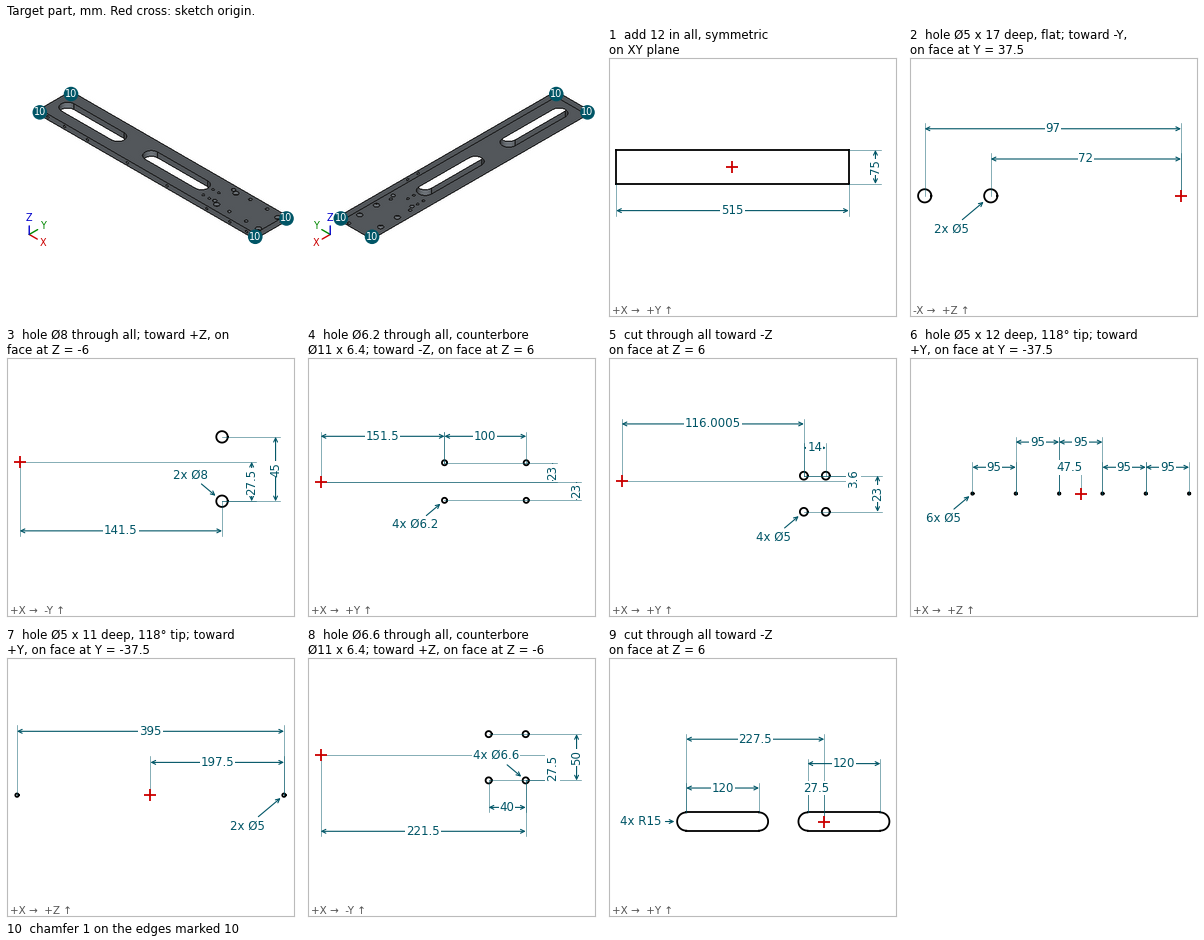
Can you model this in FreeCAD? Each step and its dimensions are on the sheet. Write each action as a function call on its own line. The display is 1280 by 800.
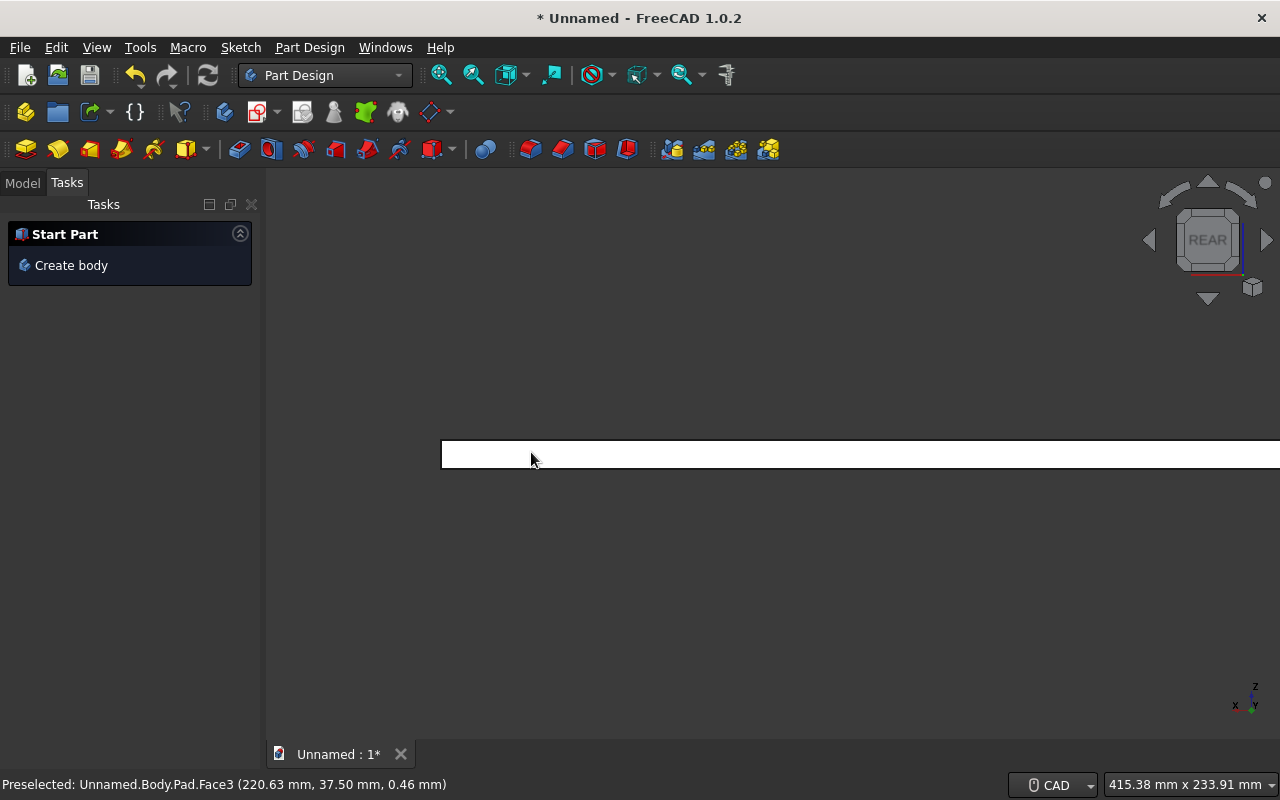
click(530, 454)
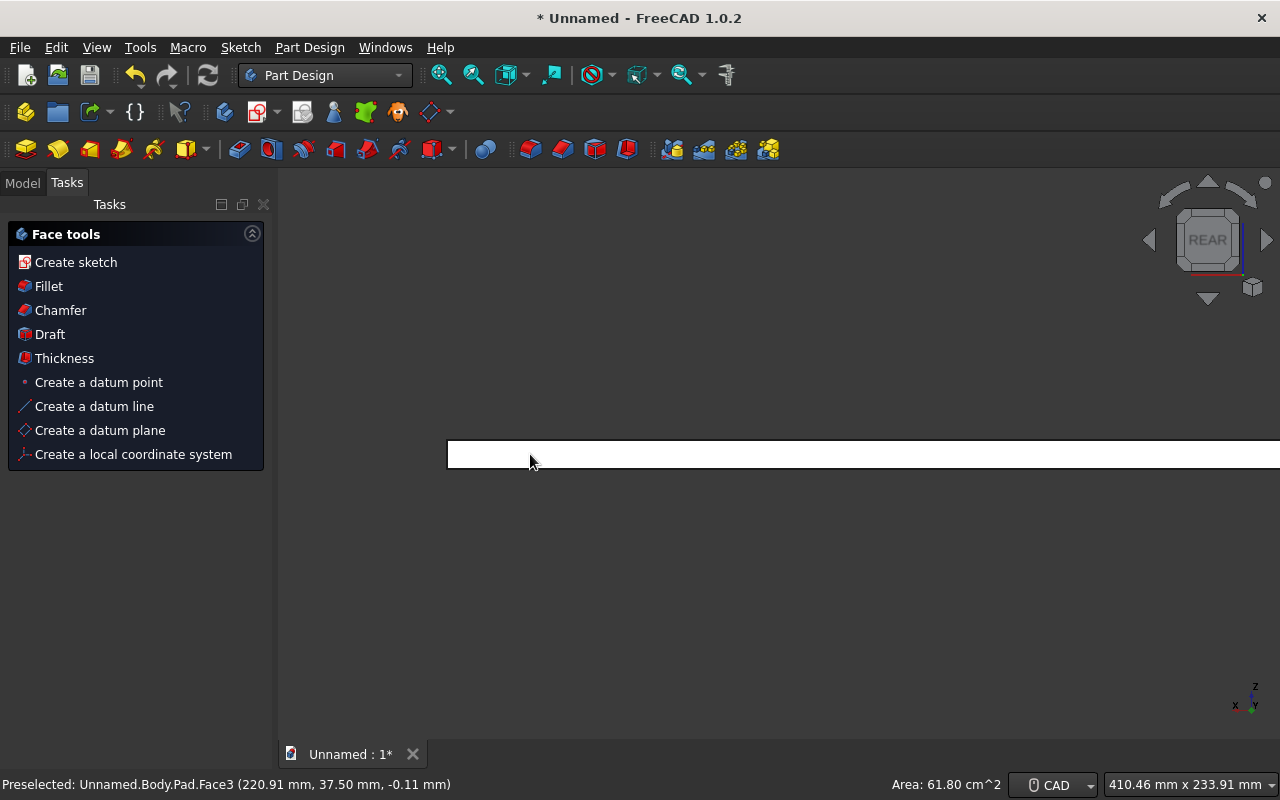
click(258, 112)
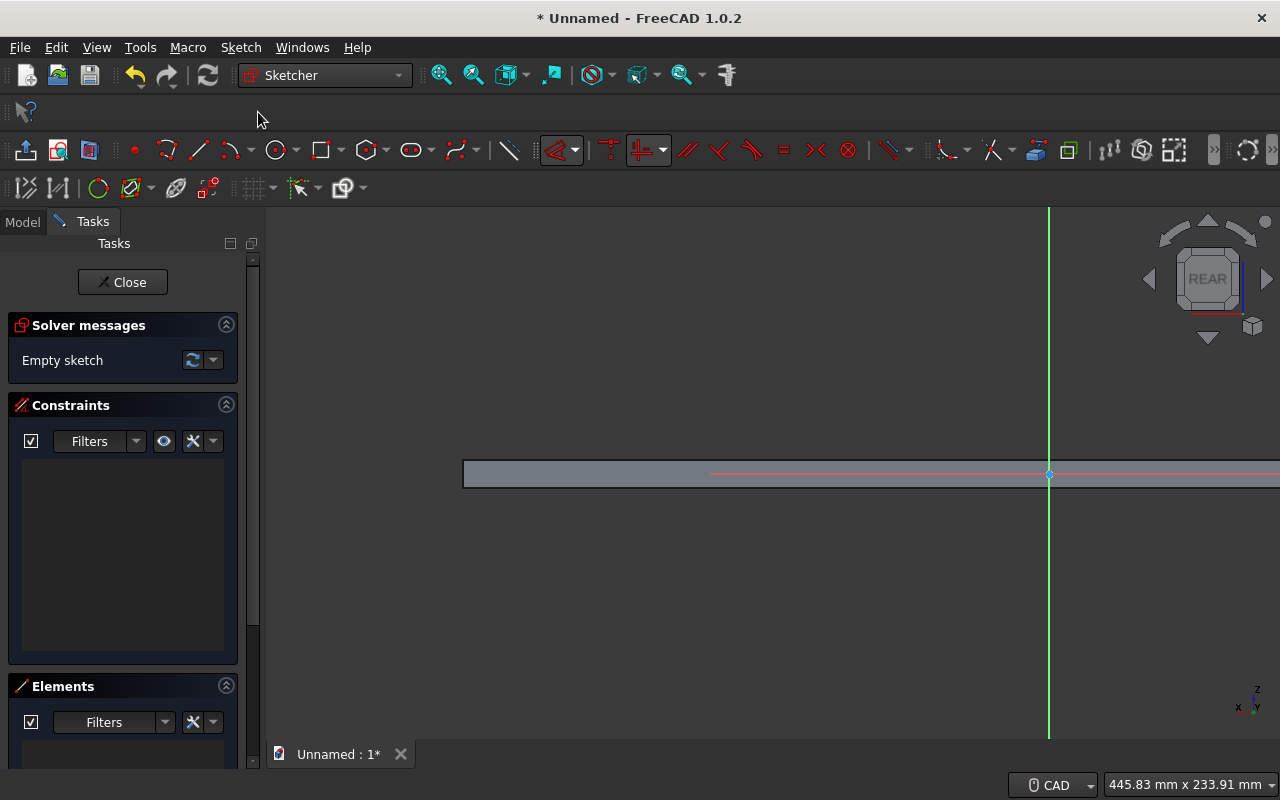
scroll(876, 474, up, 11)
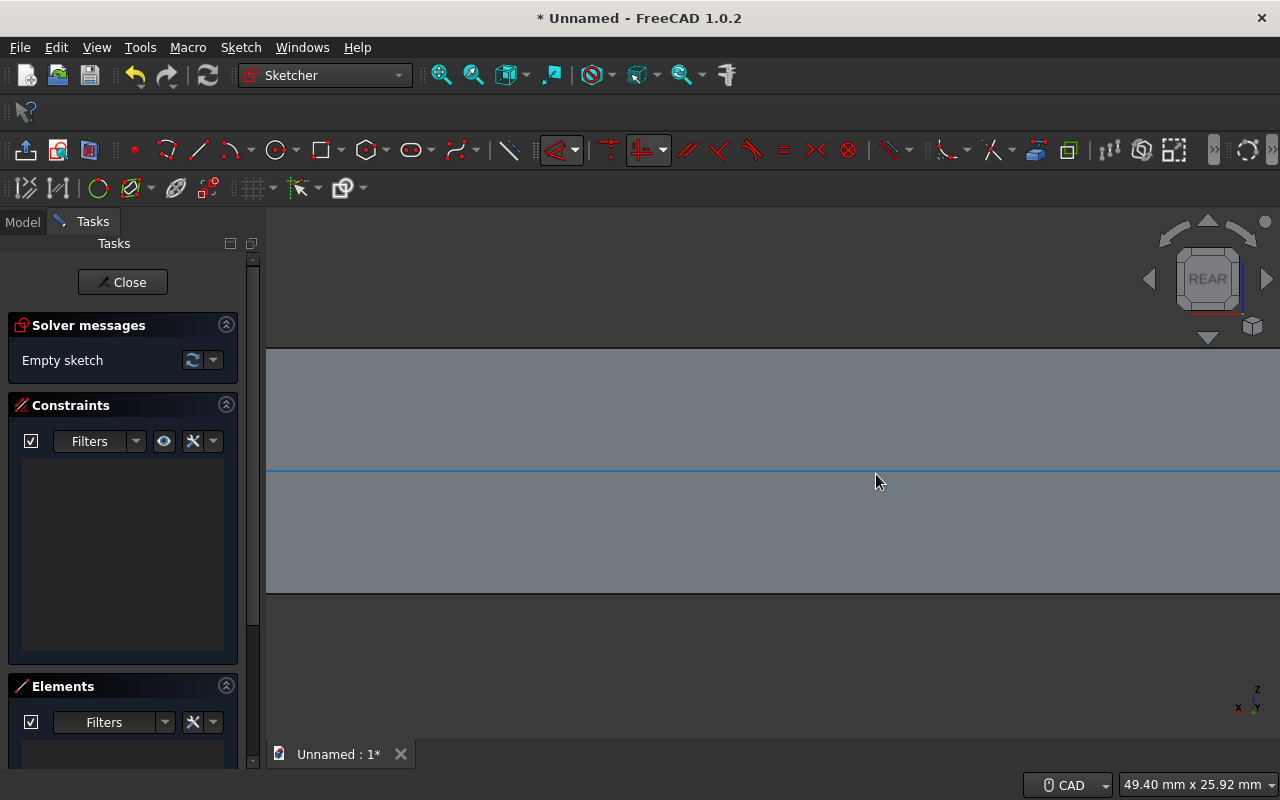
click(276, 150)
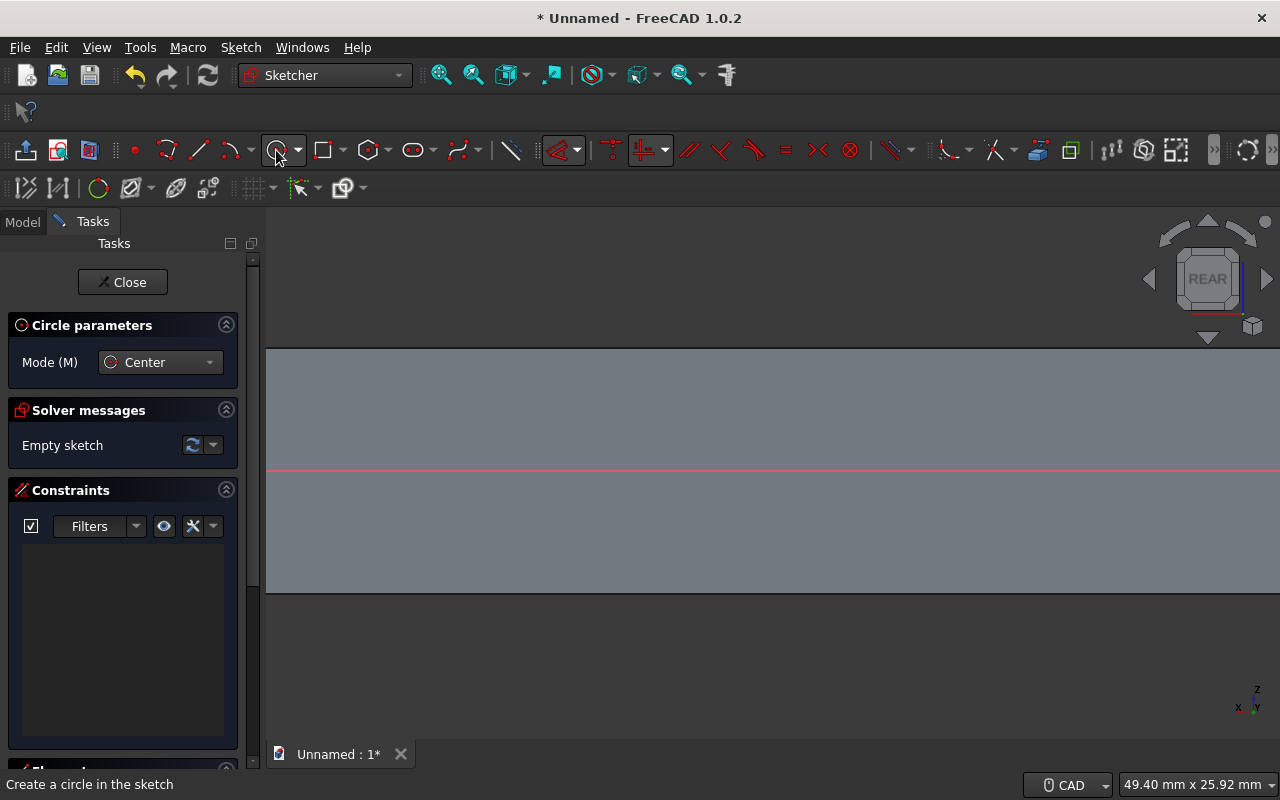
click(955, 471)
click(991, 435)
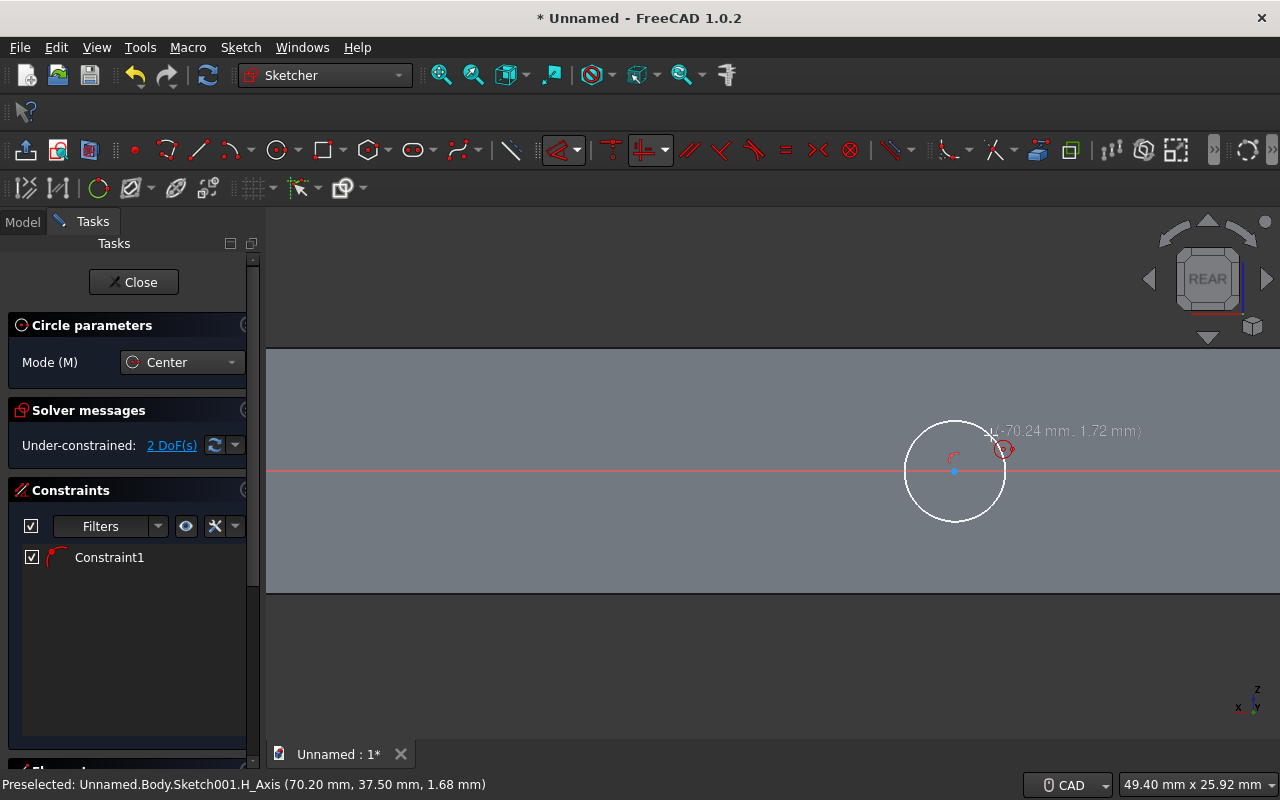
click(442, 471)
click(478, 435)
key(Escape)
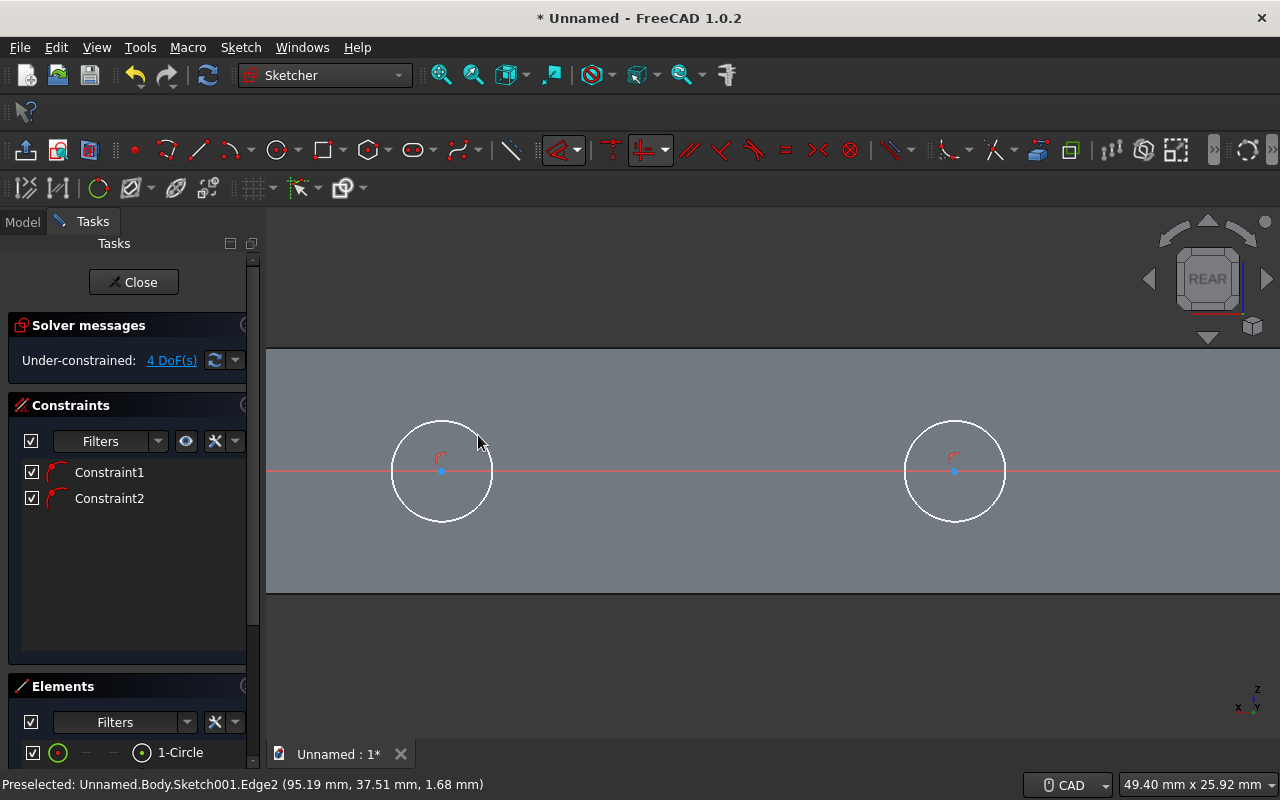
click(991, 436)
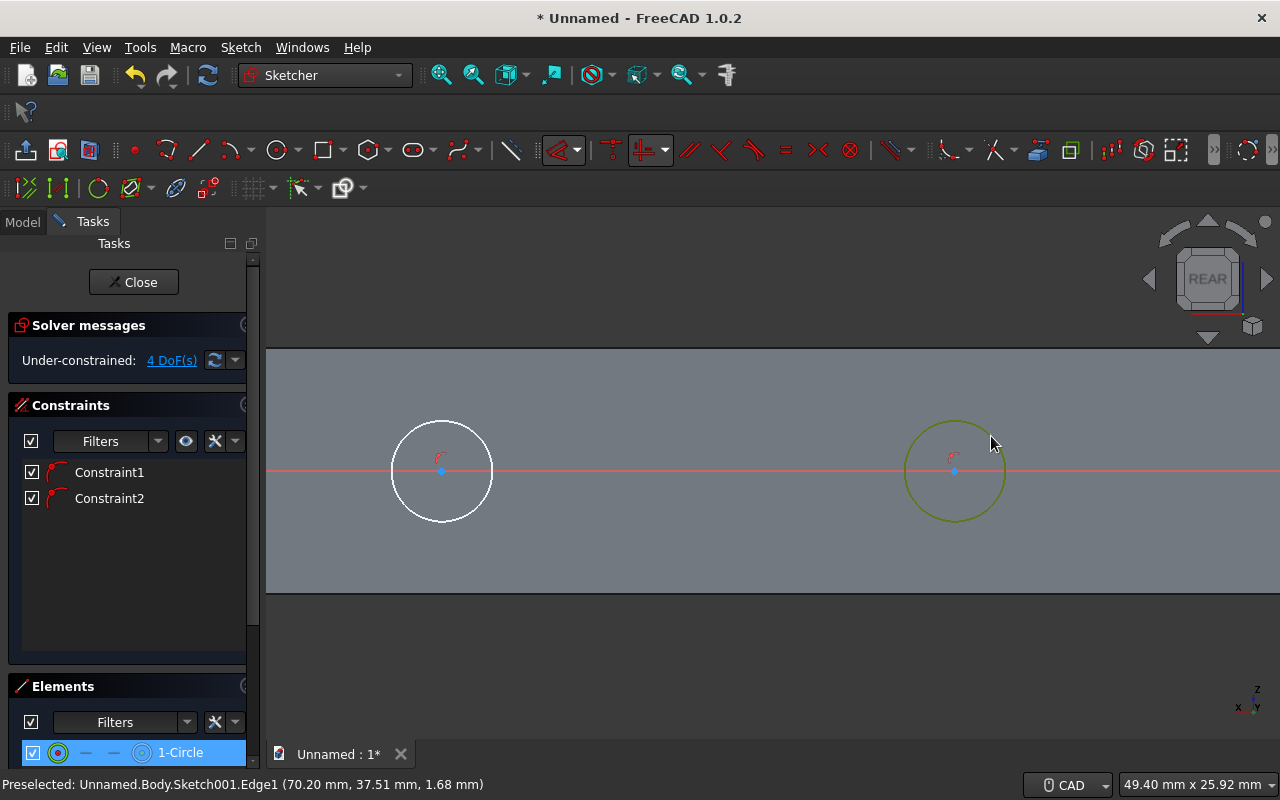
click(478, 436)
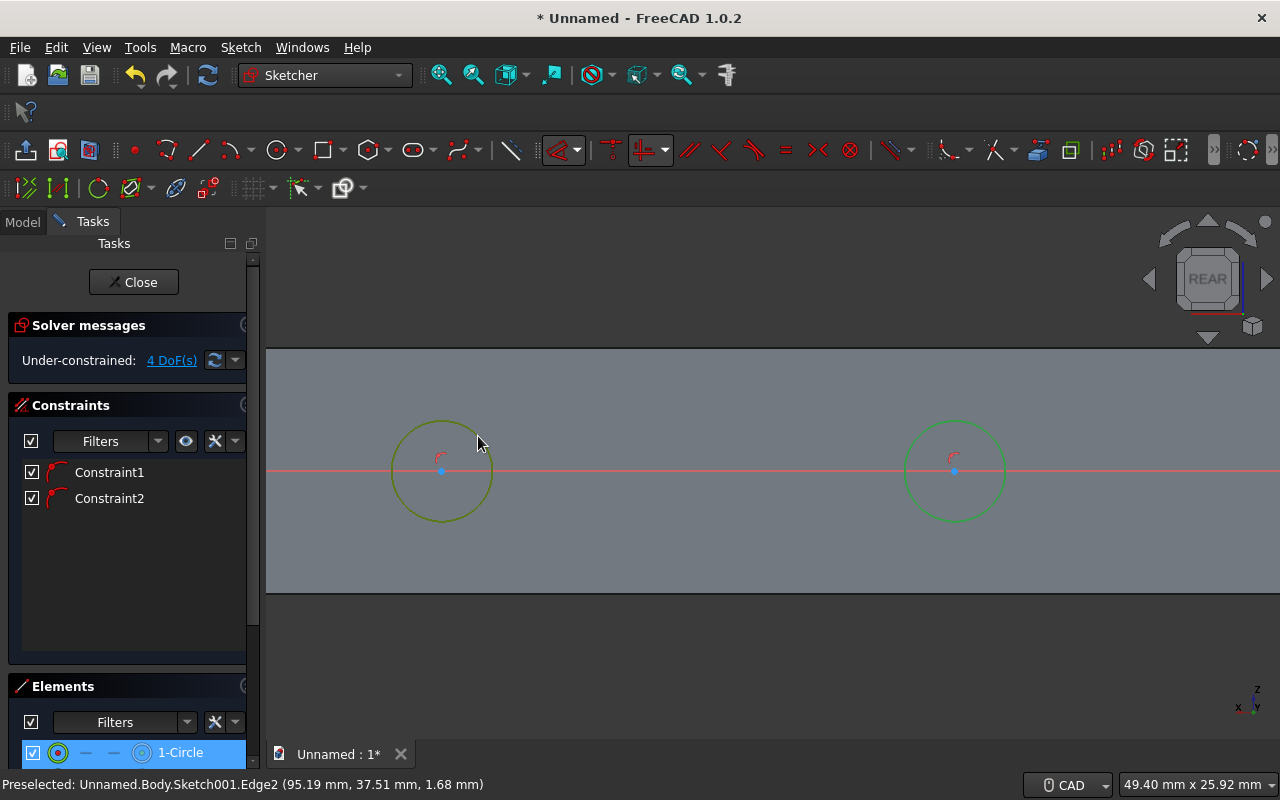
key(e)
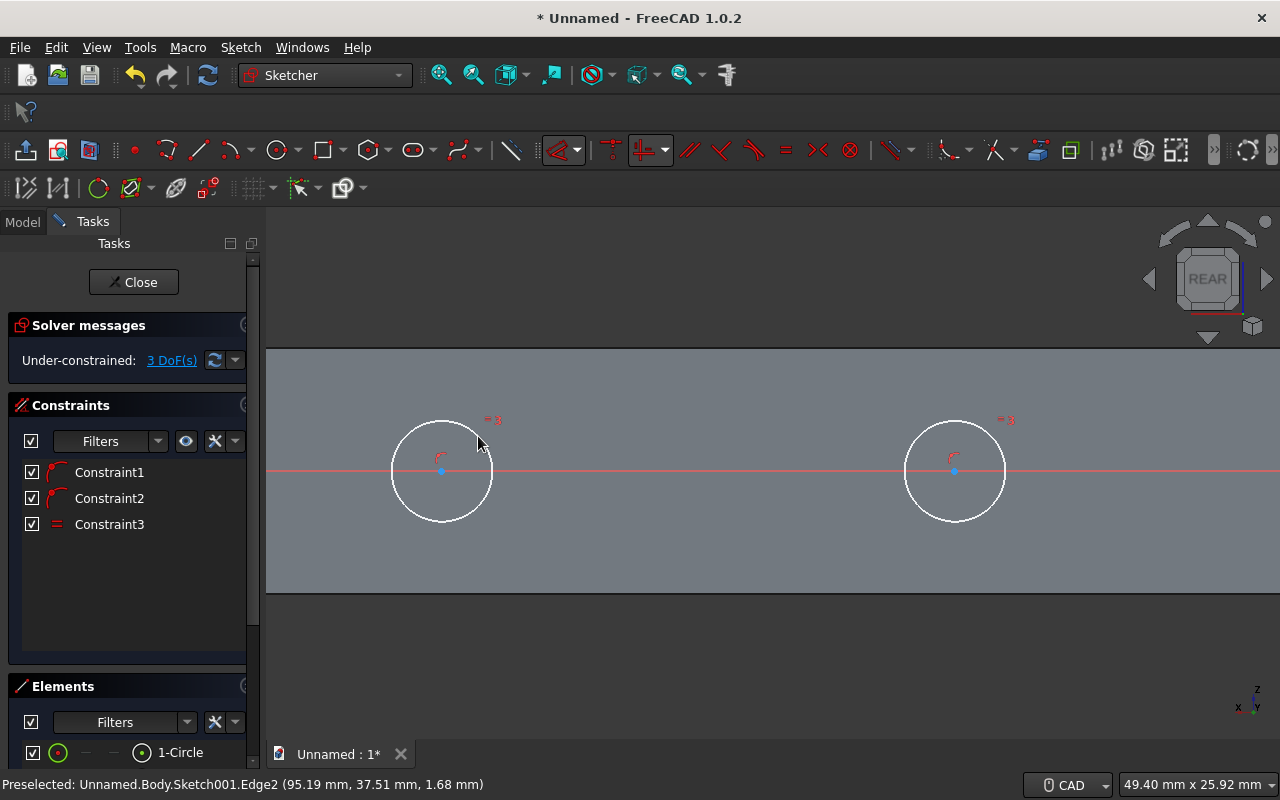
key(d)